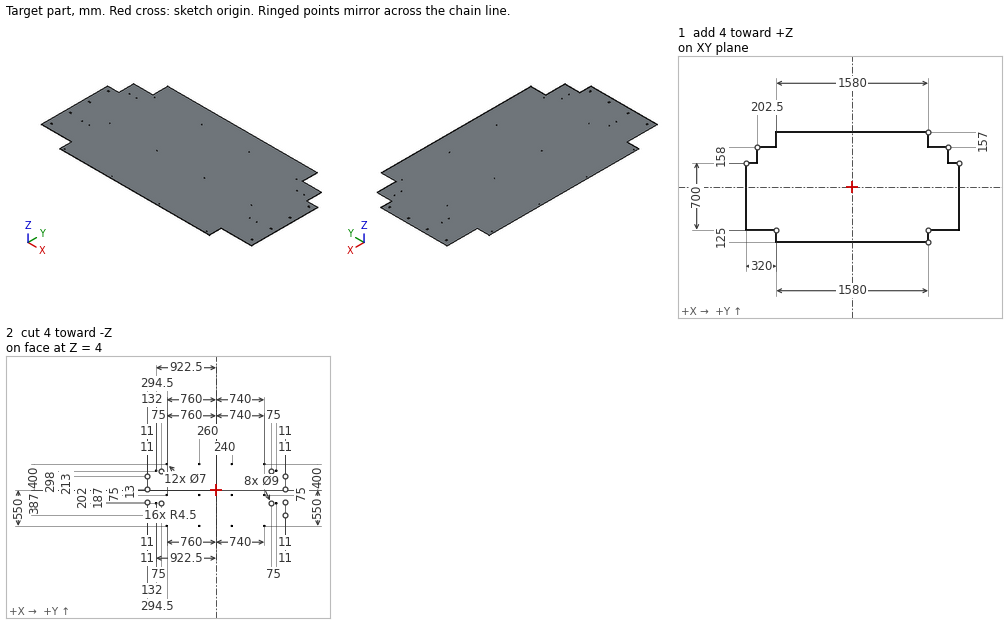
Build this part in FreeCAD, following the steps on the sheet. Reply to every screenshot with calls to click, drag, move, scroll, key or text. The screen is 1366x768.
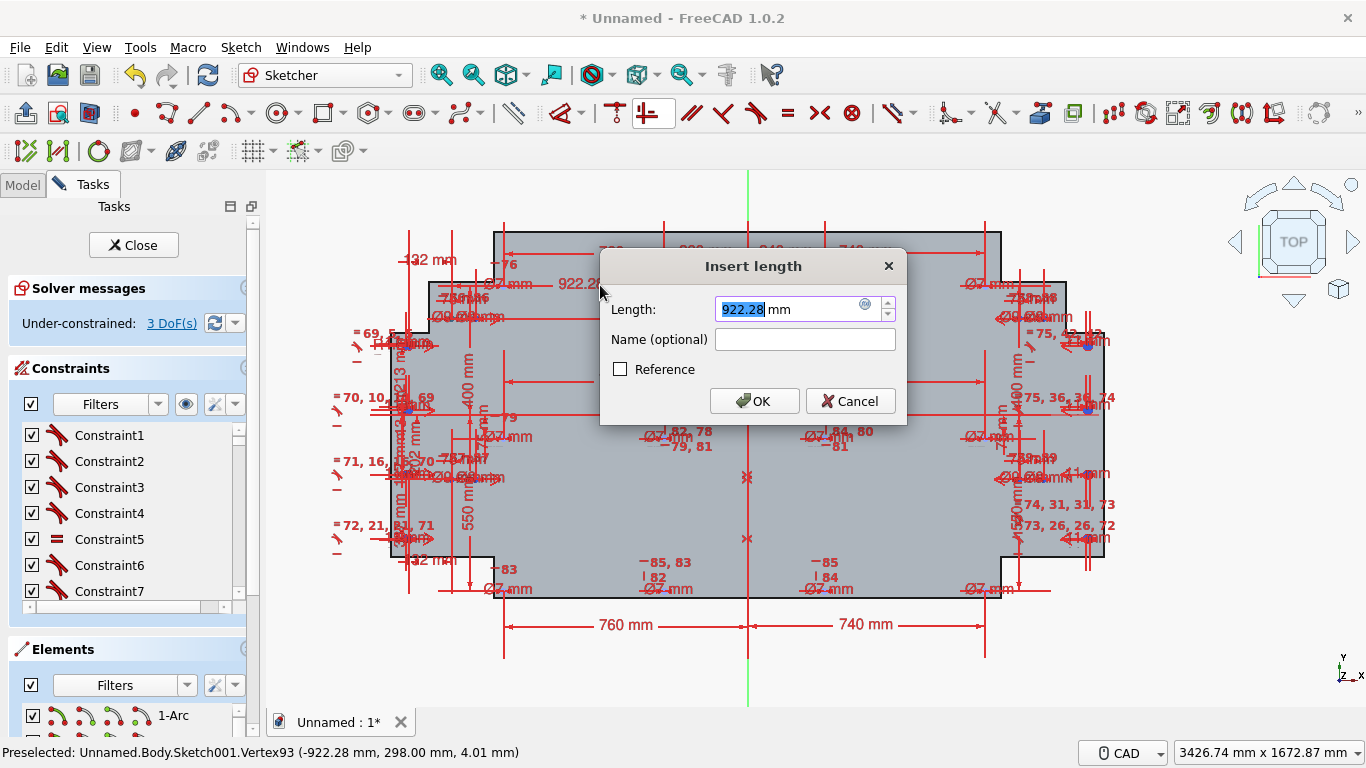
text(922.5)
key(Return)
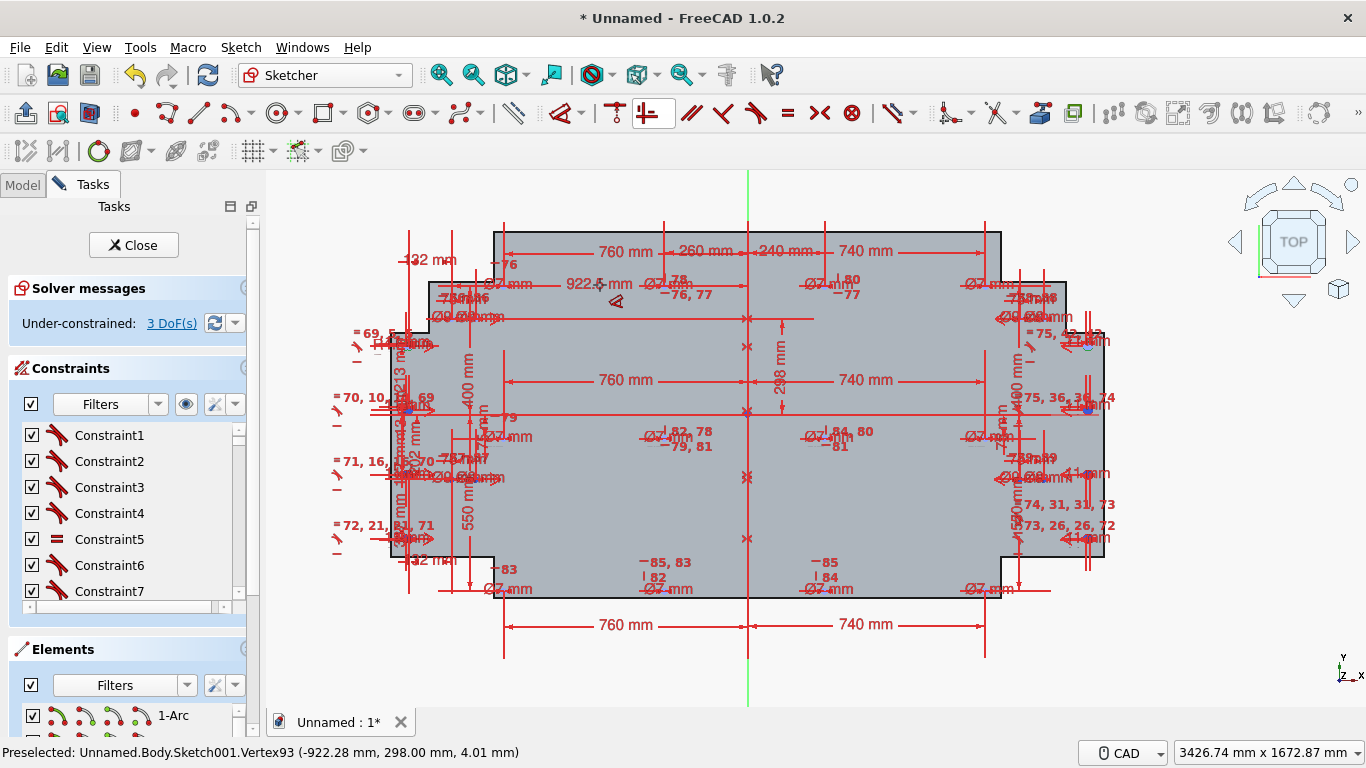
click(452, 479)
click(600, 513)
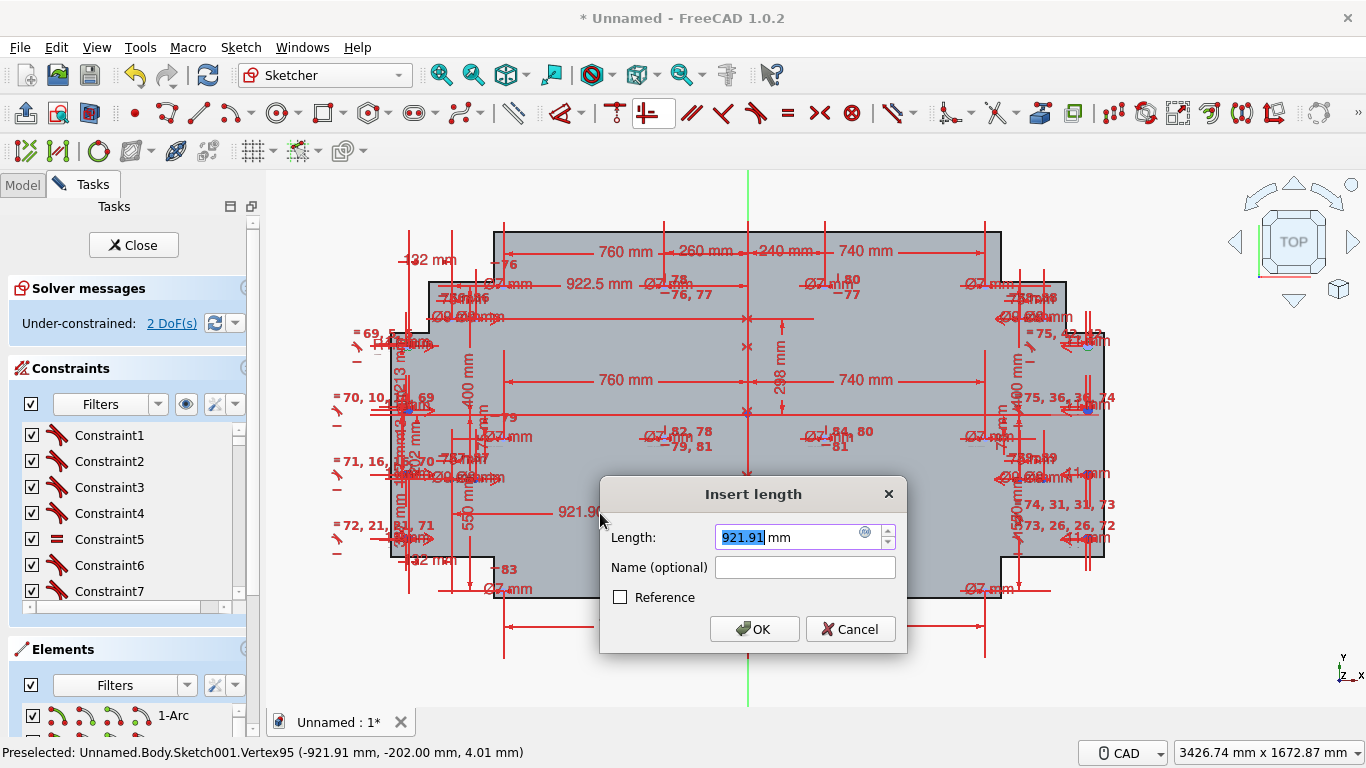
text(922.5)
key(Return)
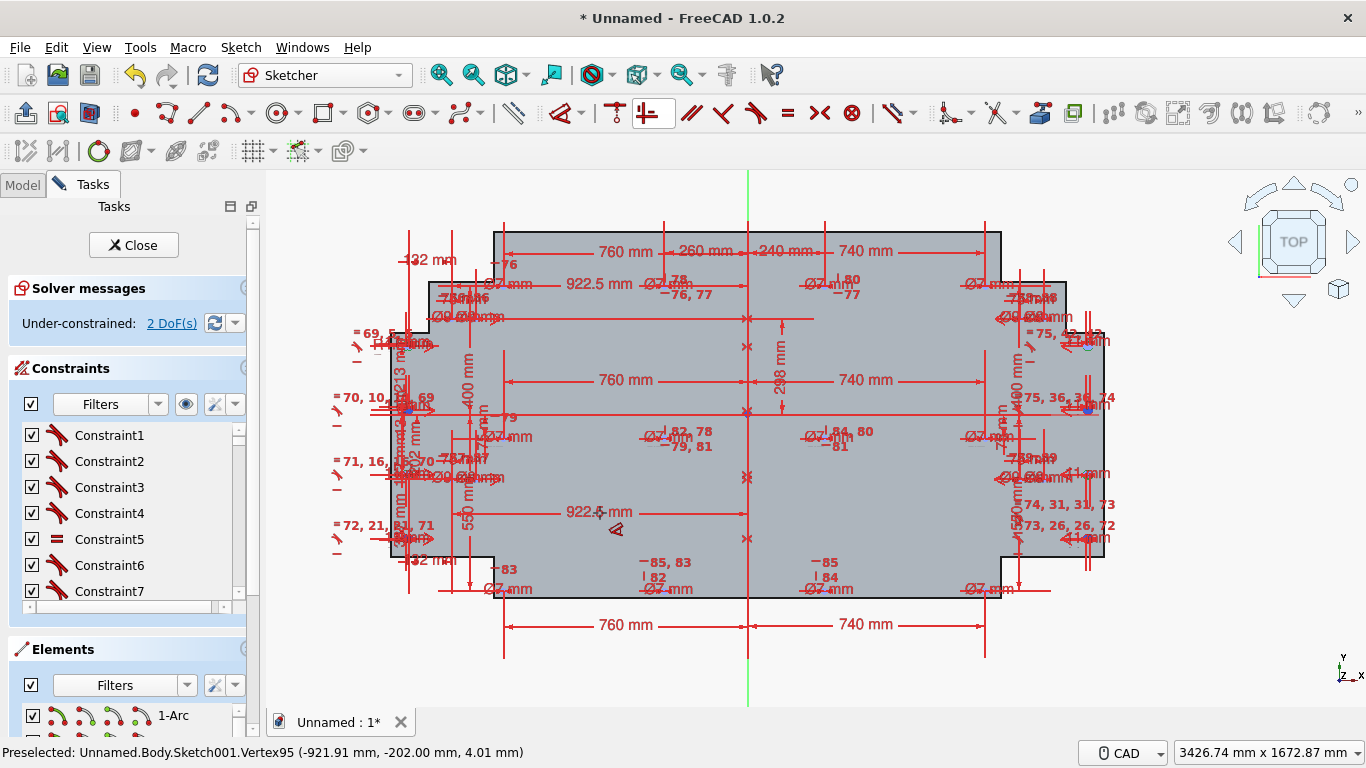
scroll(409, 412, up, 11)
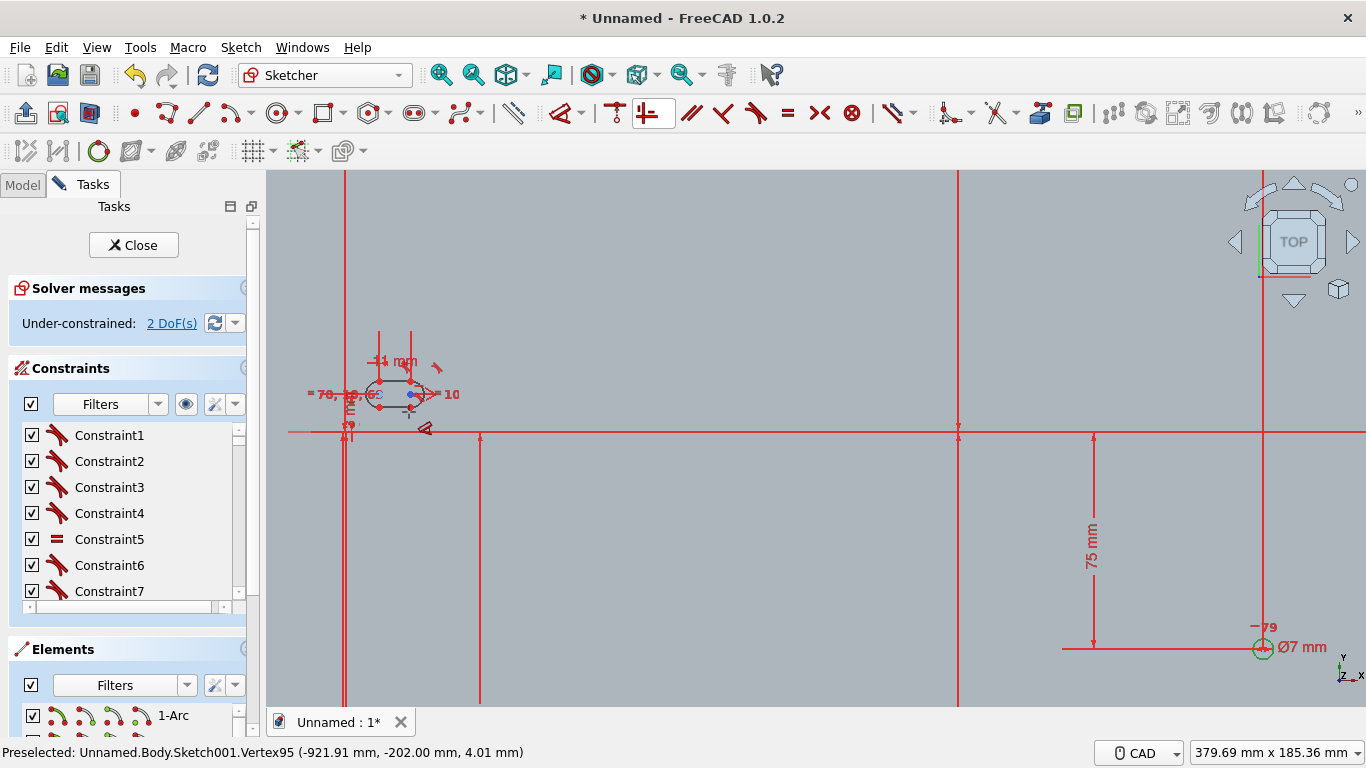
click(411, 407)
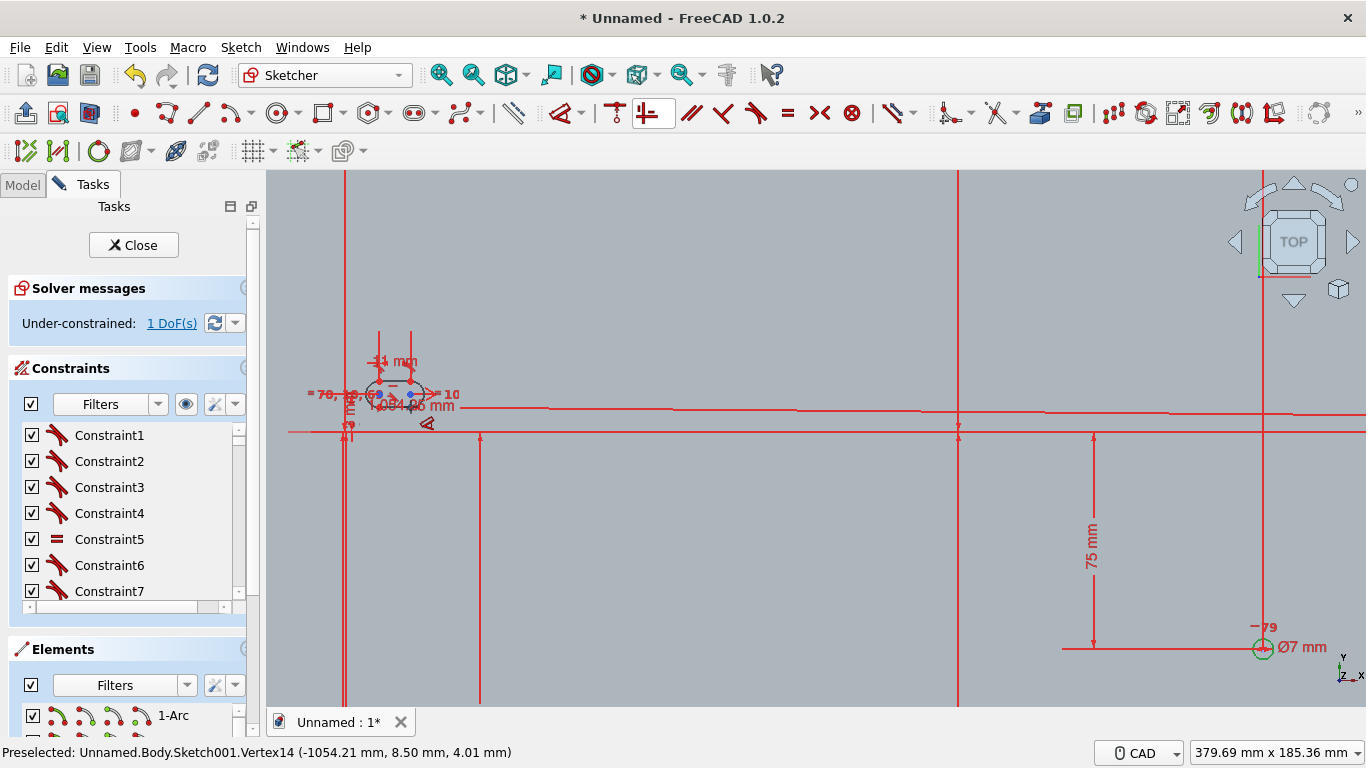
scroll(409, 412, down, 11)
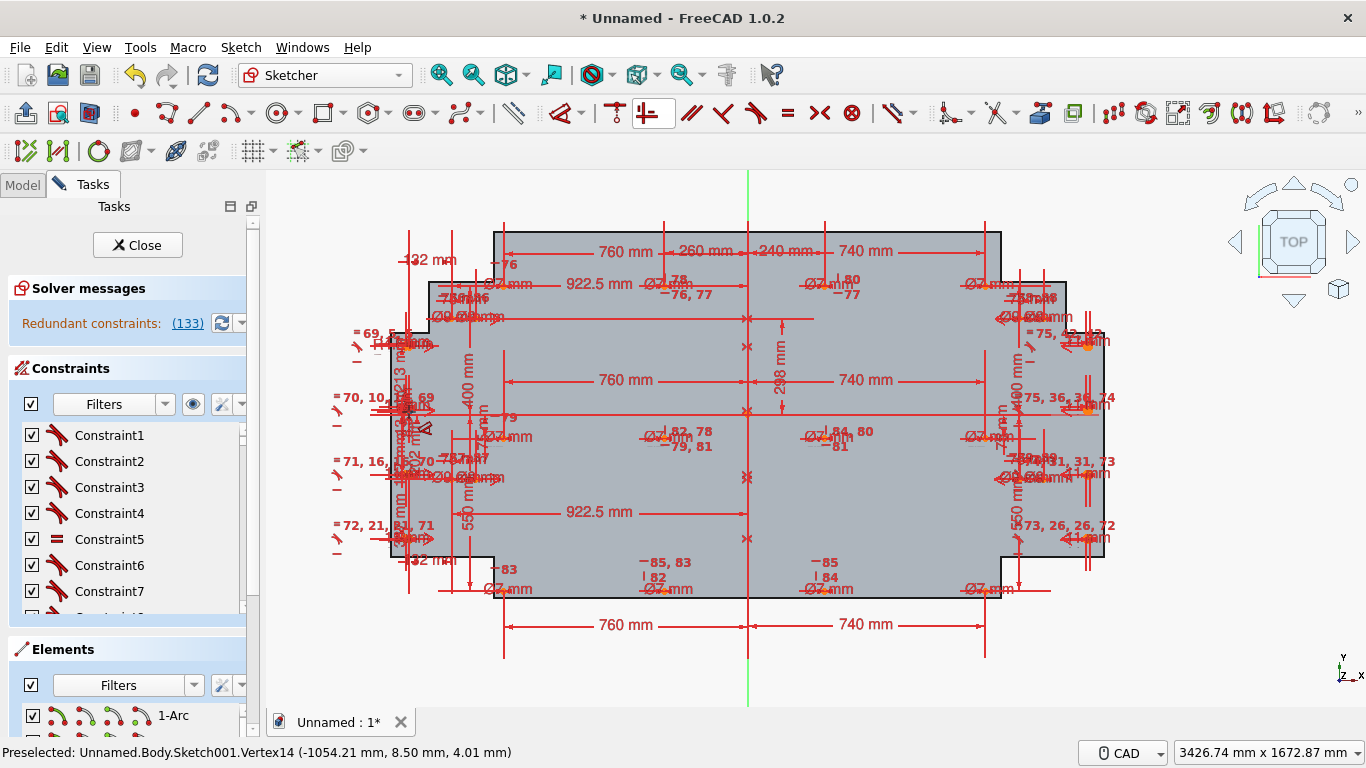
click(504, 439)
click(478, 354)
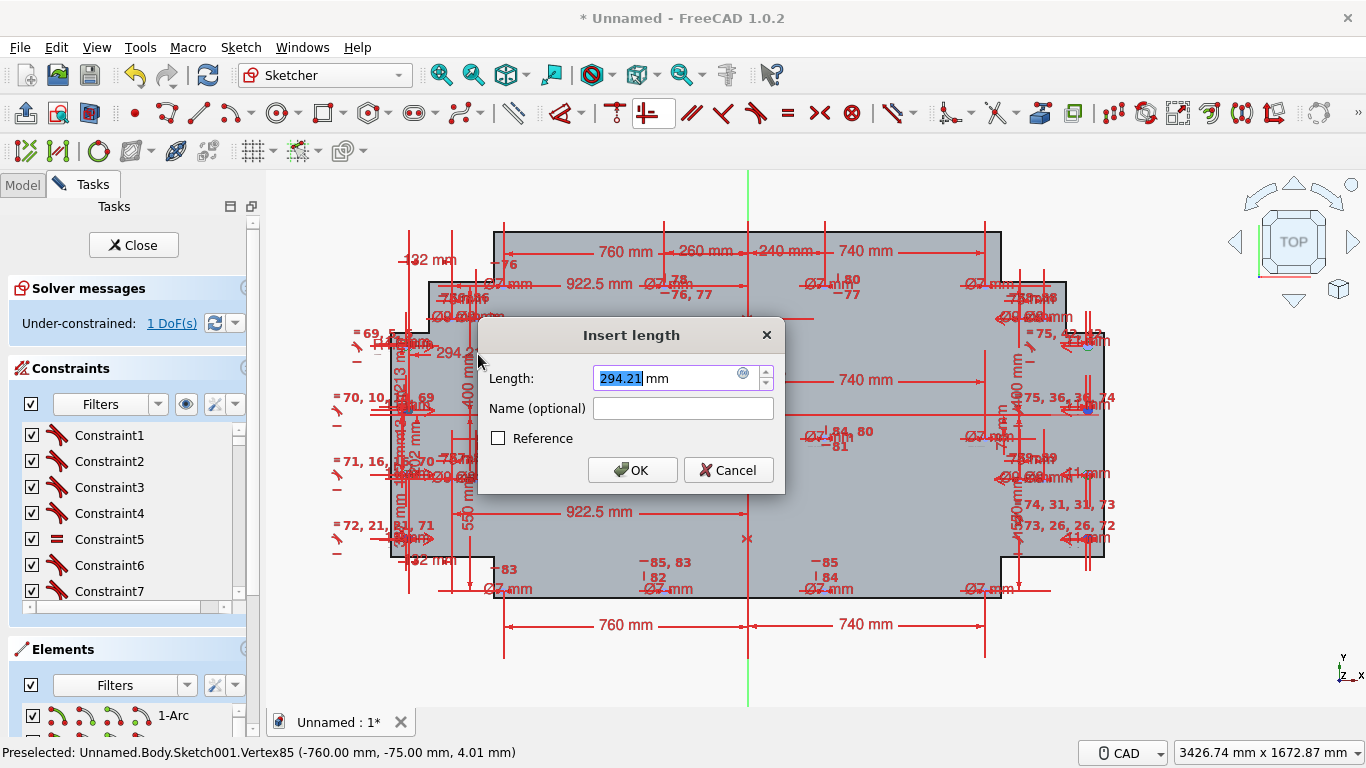
text(294.5)
key(Return)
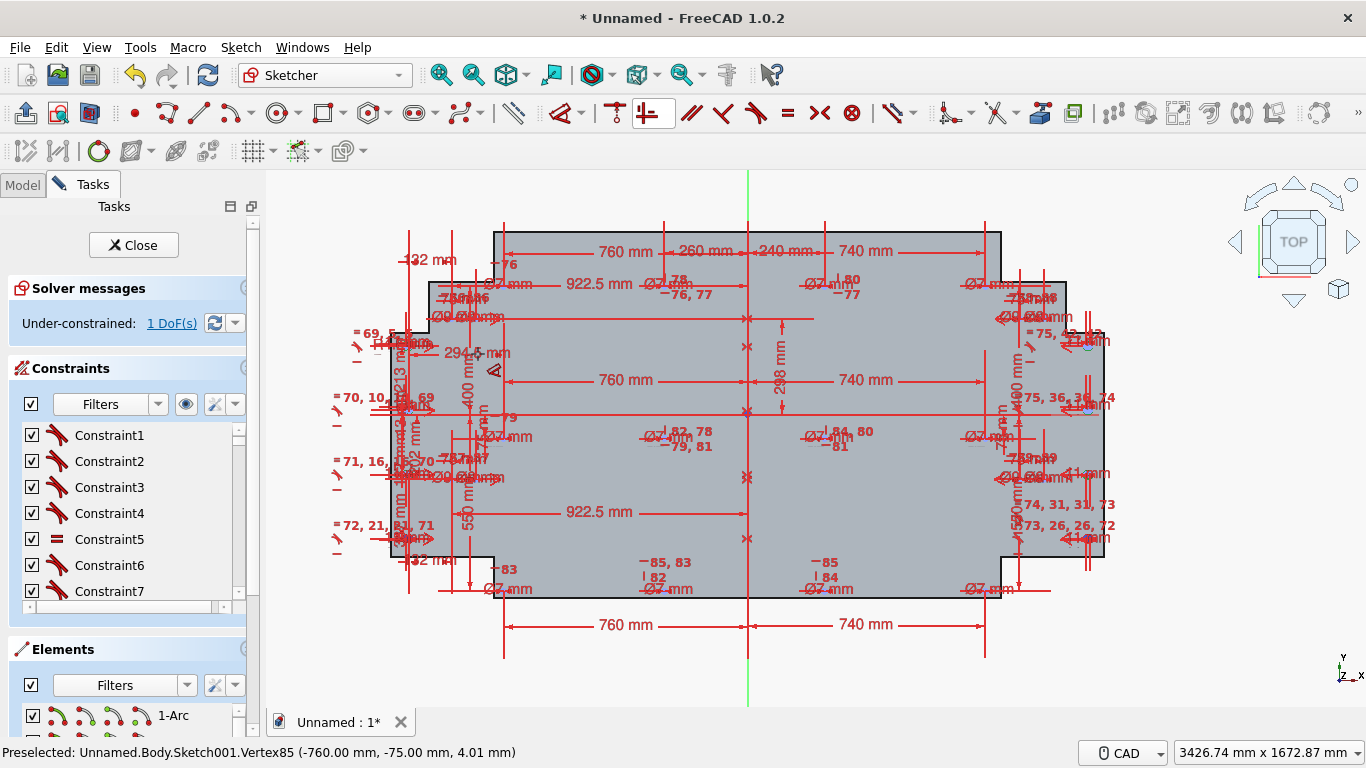
scroll(409, 540, up, 11)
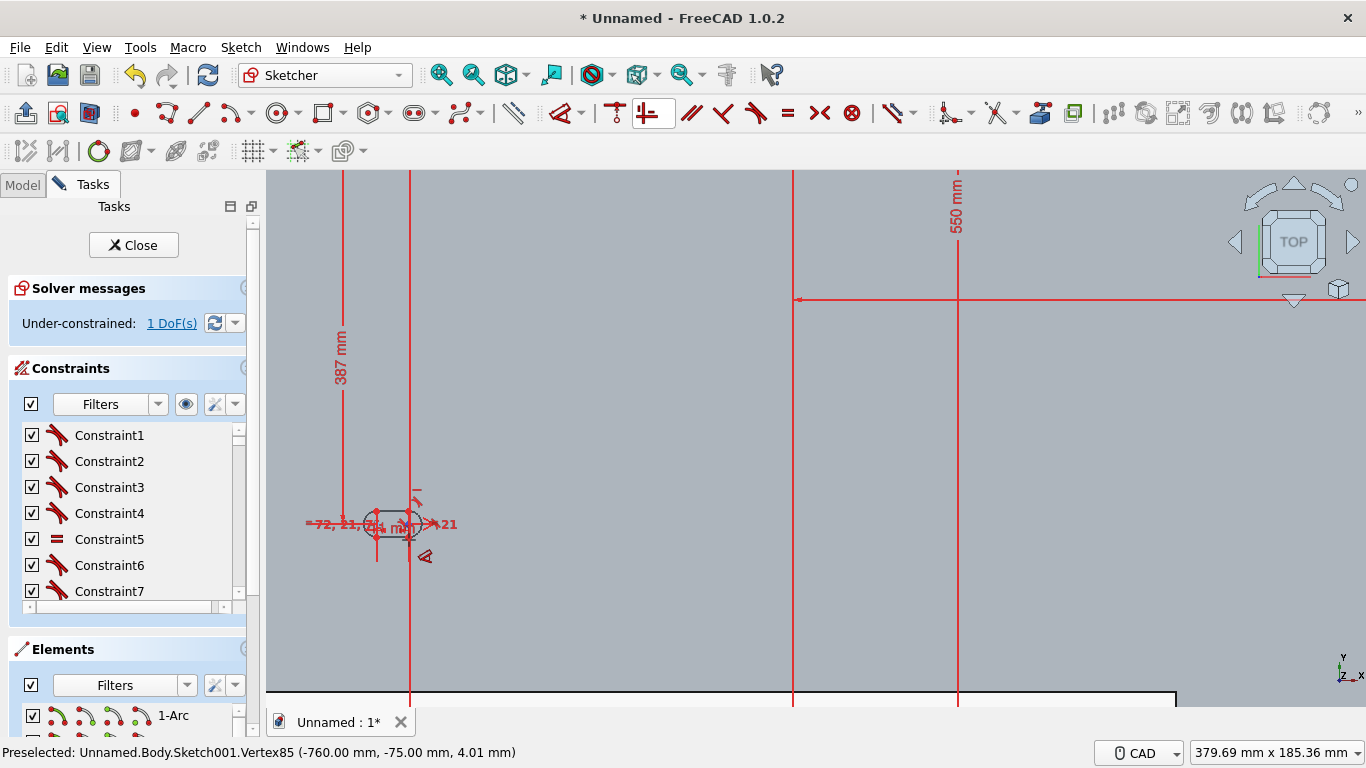
click(409, 537)